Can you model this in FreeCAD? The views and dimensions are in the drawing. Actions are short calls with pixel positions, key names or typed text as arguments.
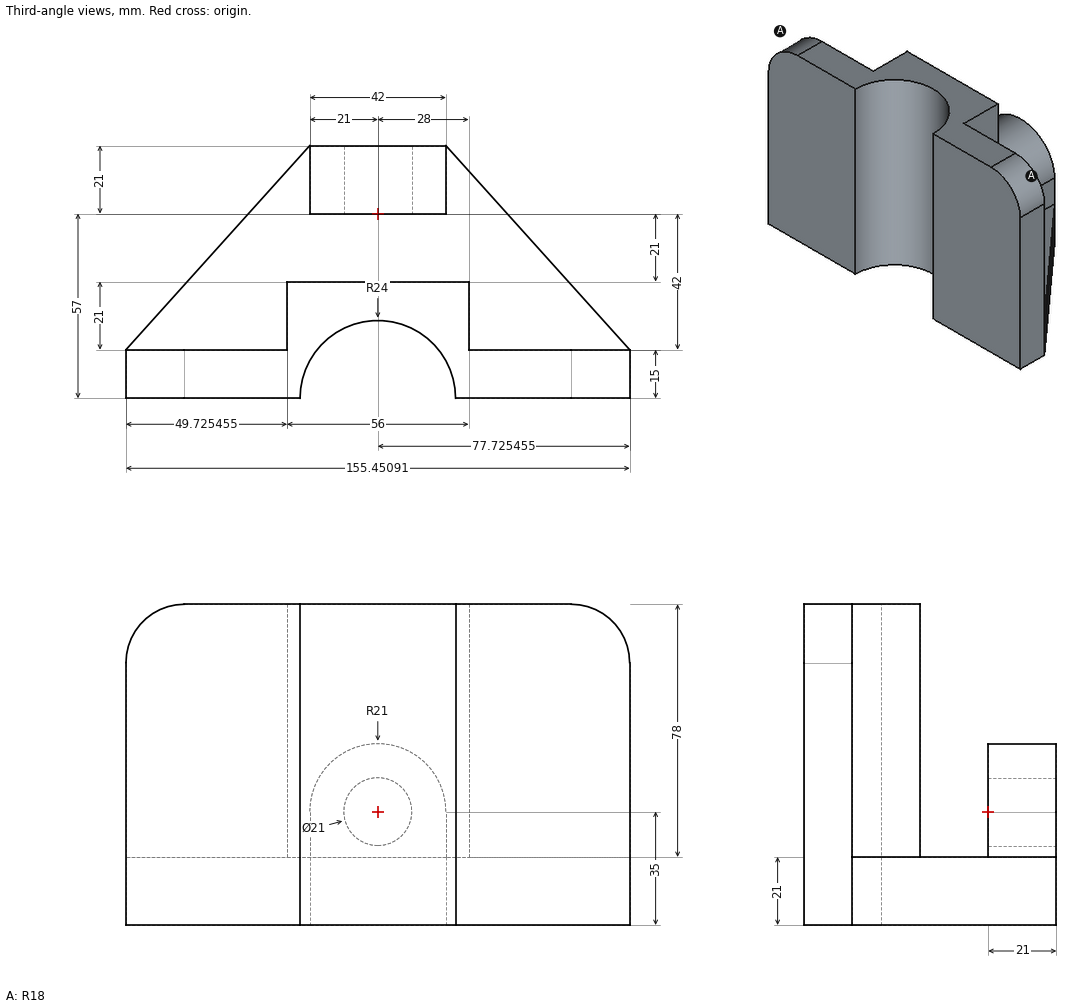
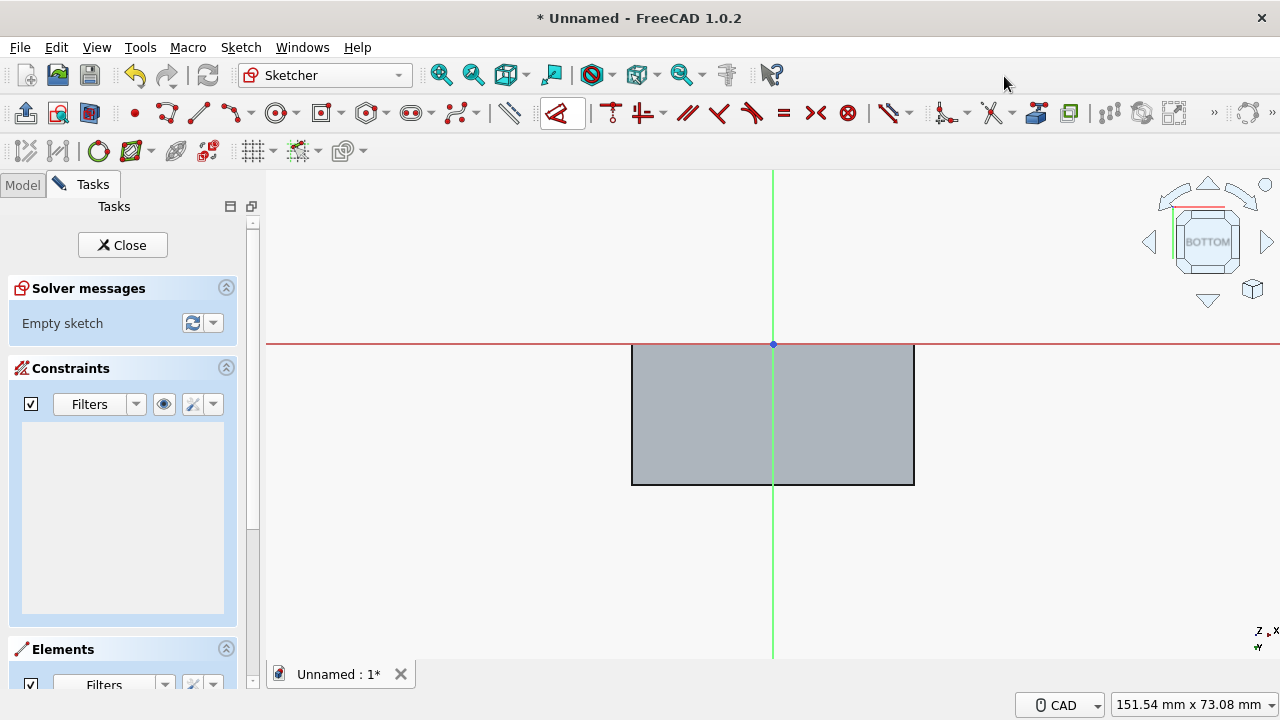
scroll(621, 631, down, 3)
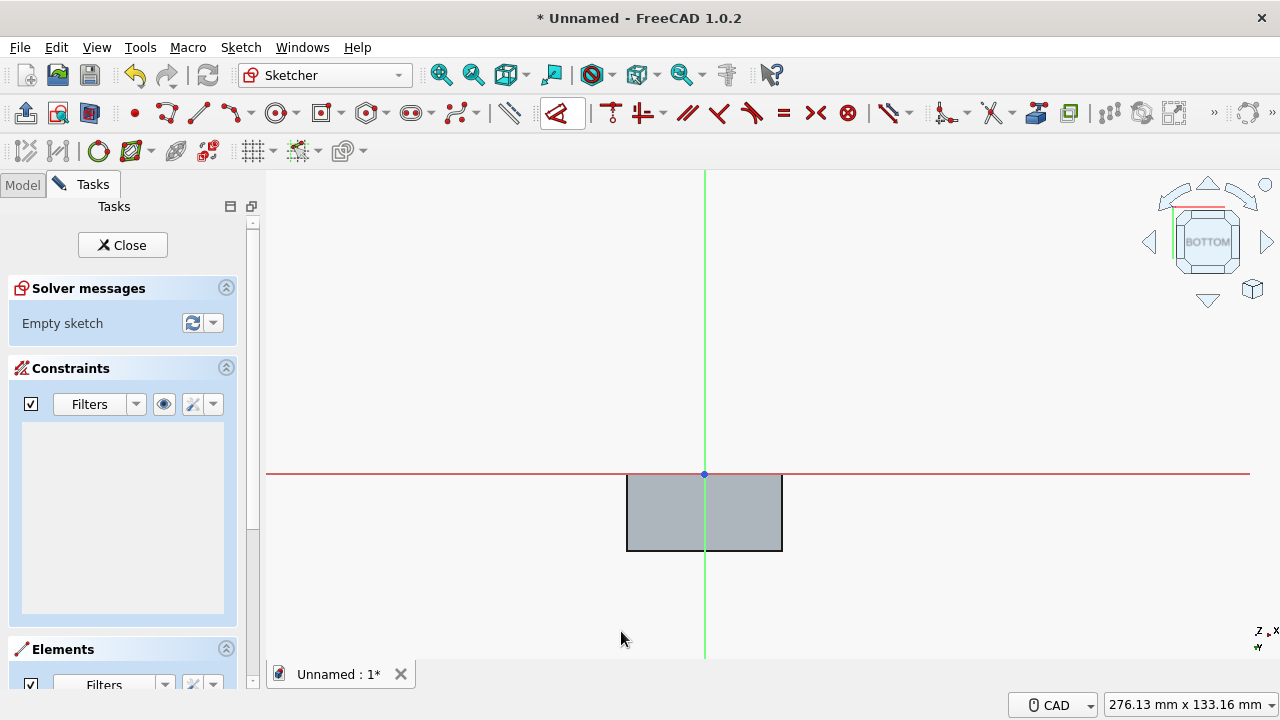
click(168, 114)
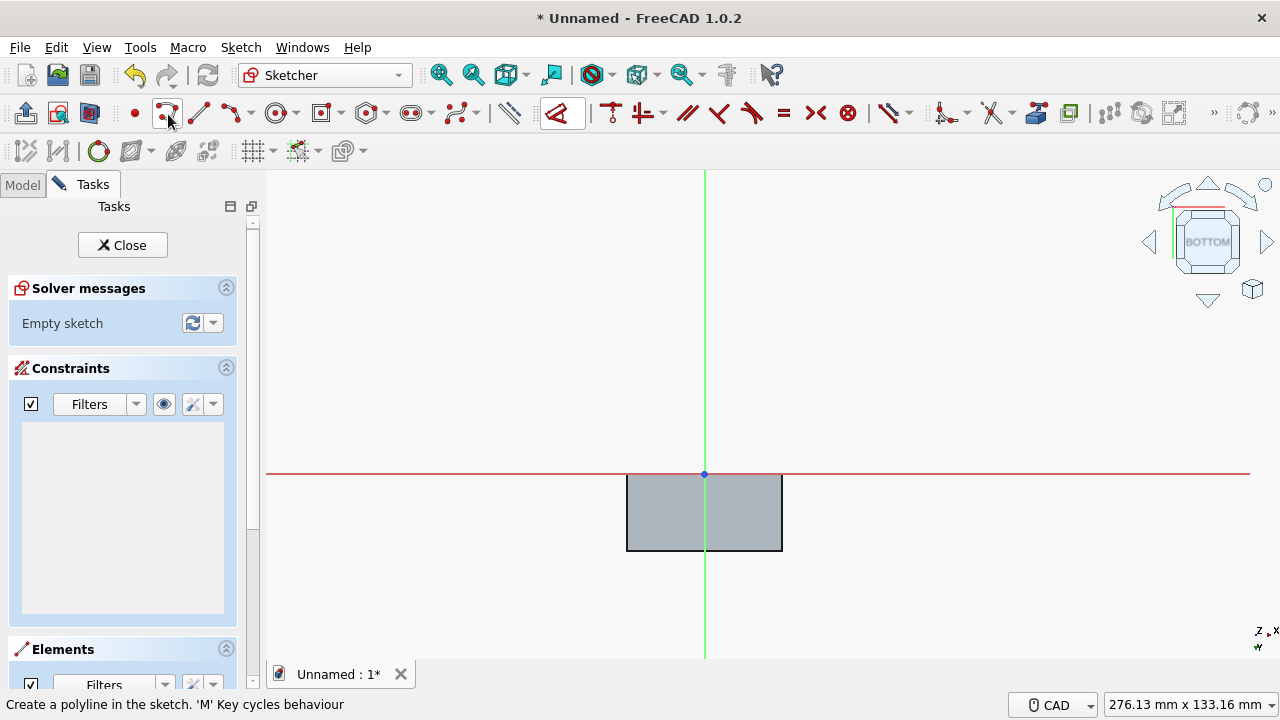
click(627, 551)
click(782, 551)
click(990, 320)
click(990, 265)
click(419, 265)
click(419, 320)
click(627, 552)
key(Escape)
key(Escape)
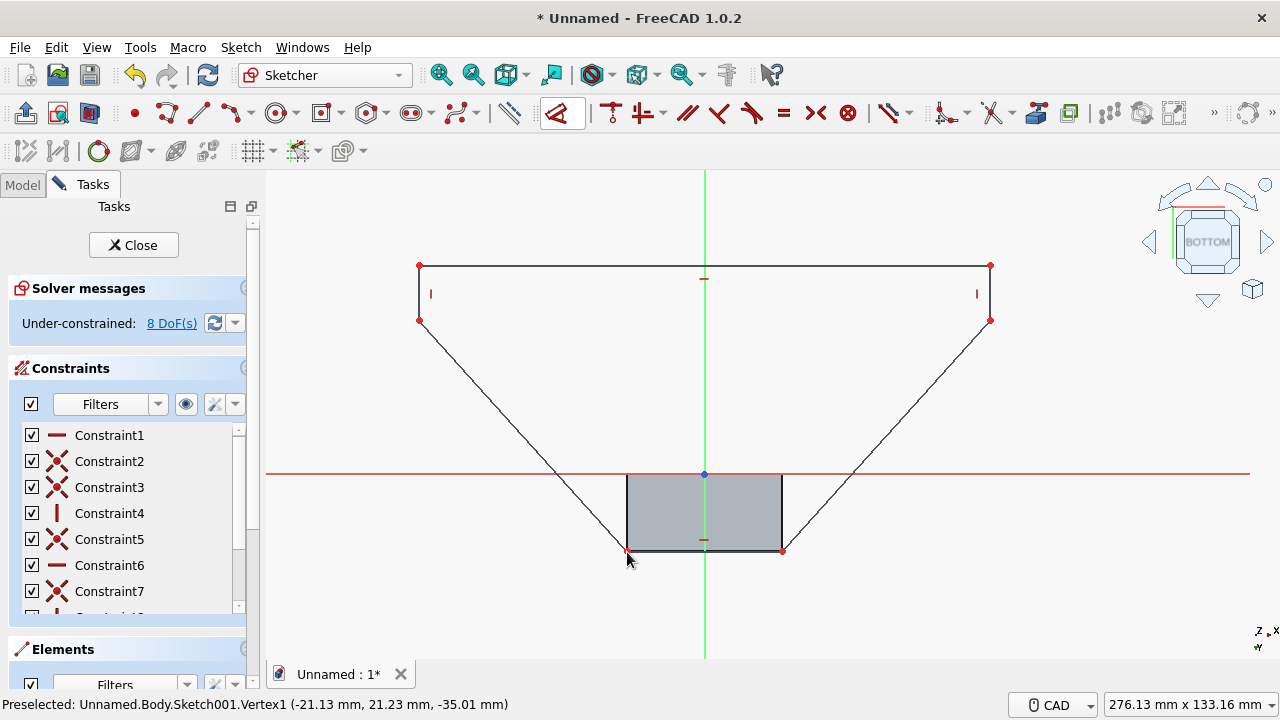
click(673, 552)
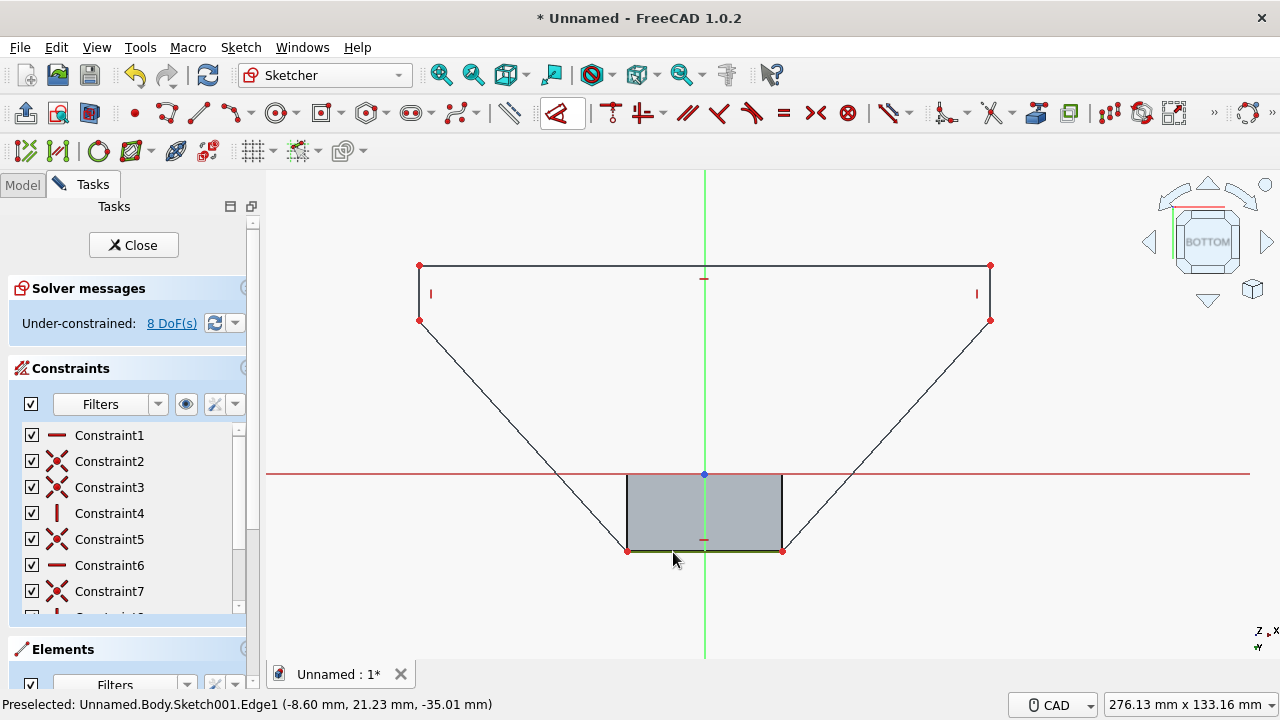
click(580, 114)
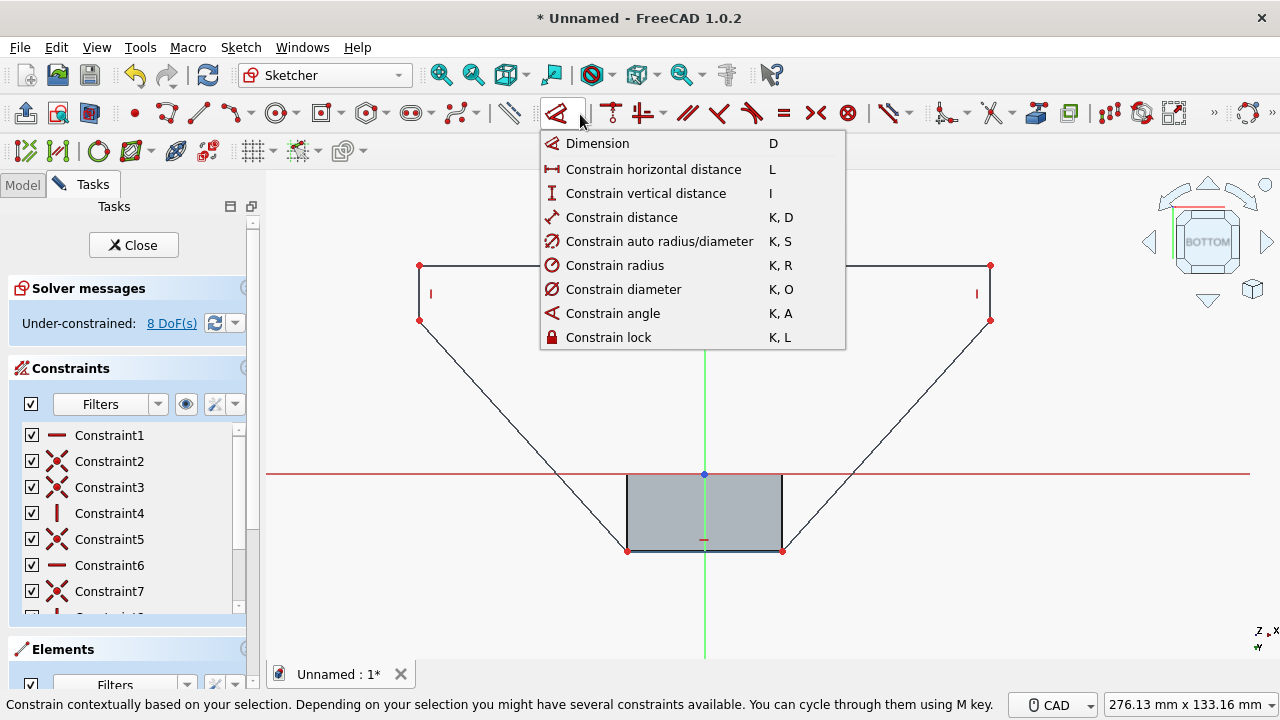
click(693, 169)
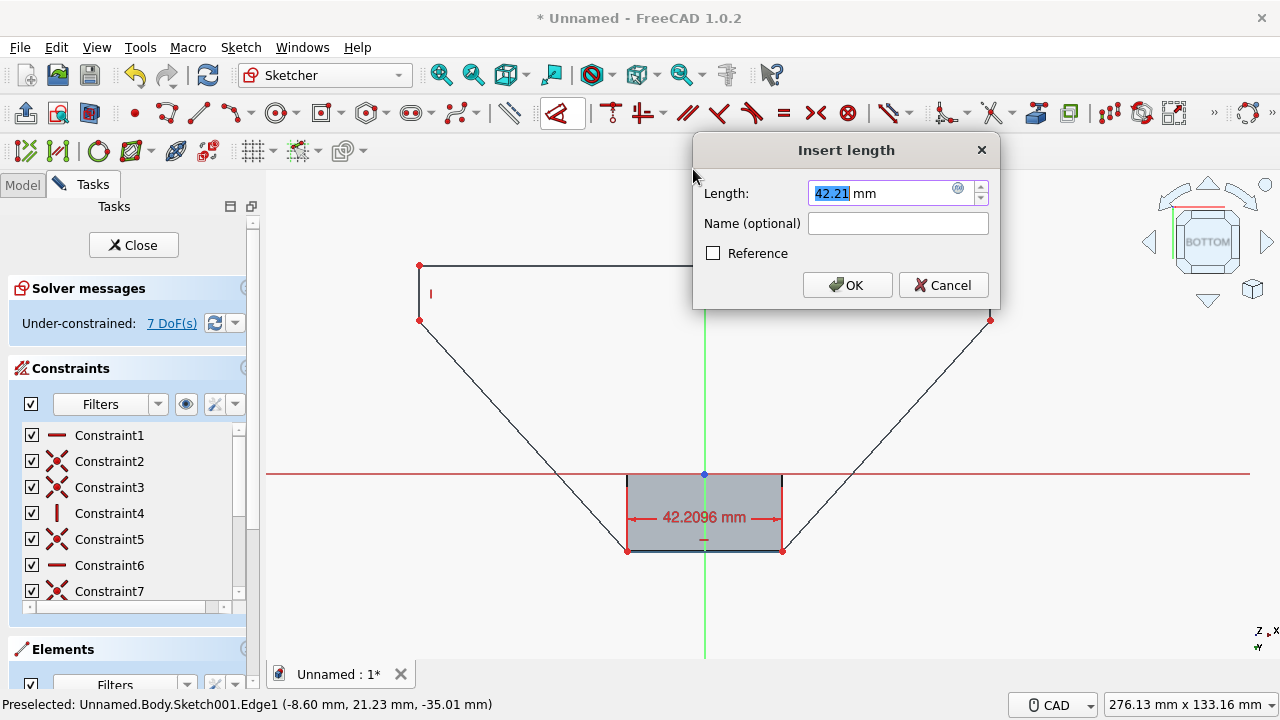
text(42)
key(Return)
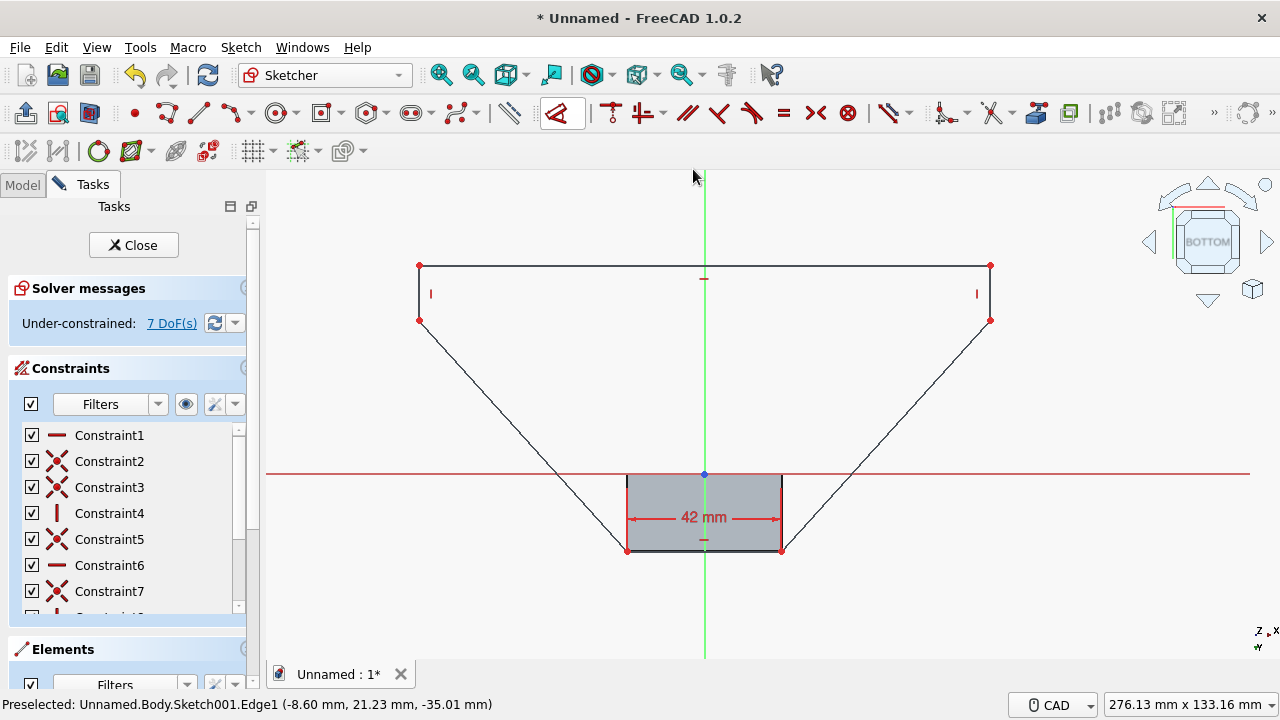
click(990, 305)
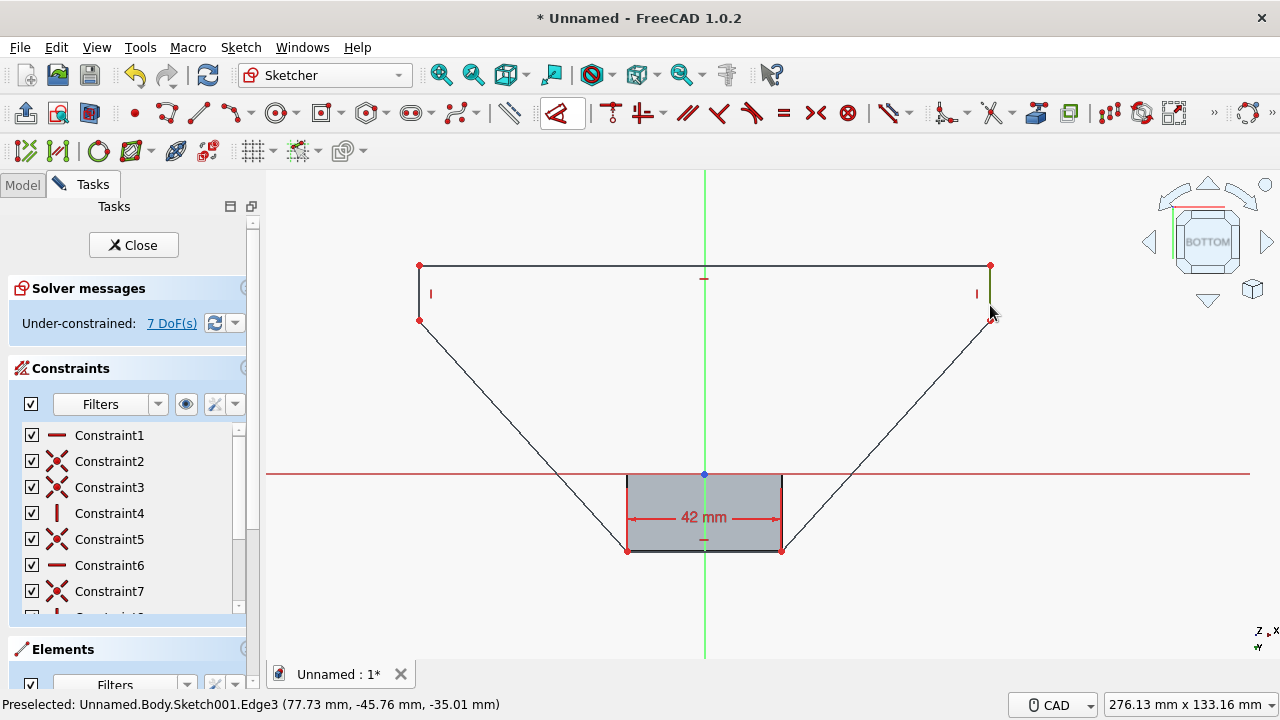
click(580, 114)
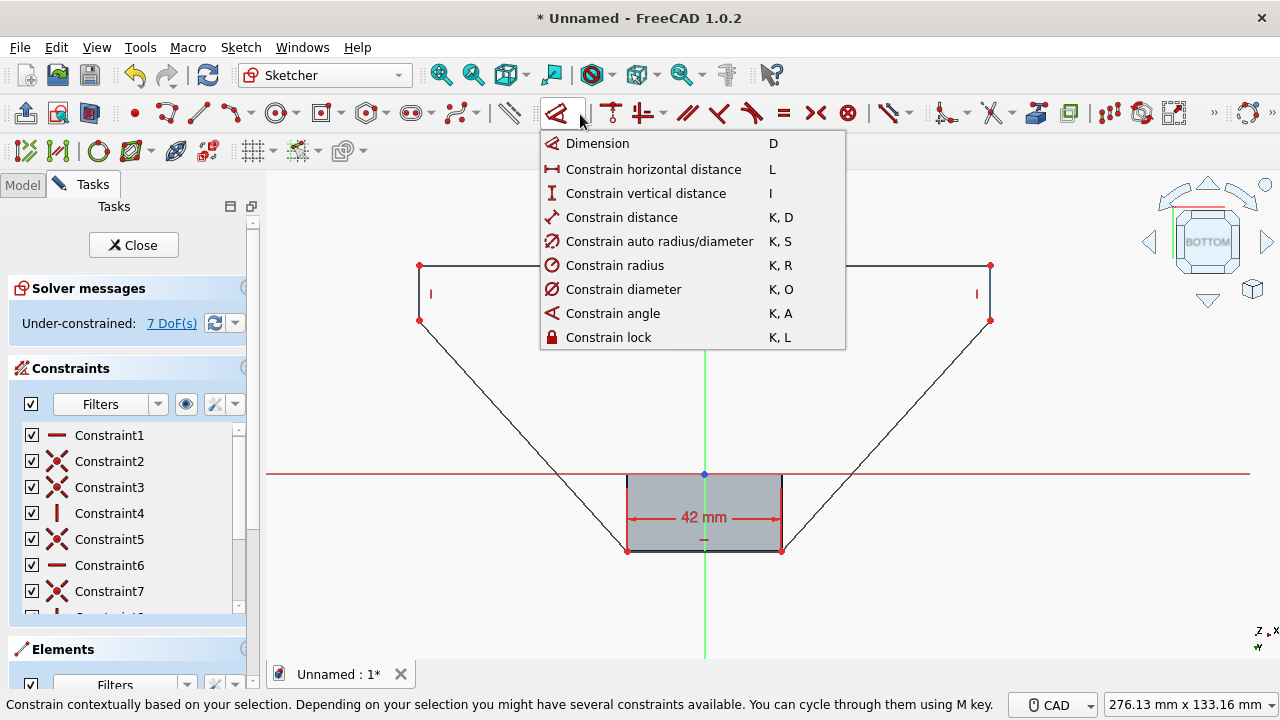
click(693, 193)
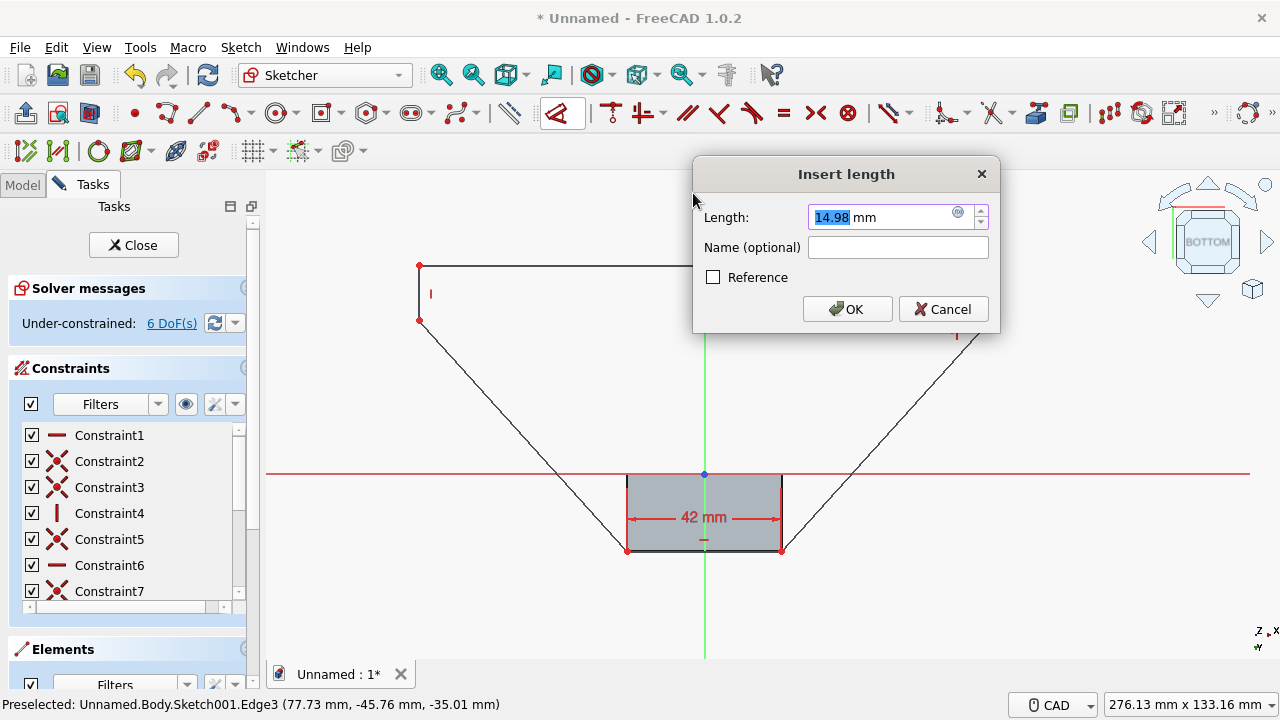
text(15)
key(Return)